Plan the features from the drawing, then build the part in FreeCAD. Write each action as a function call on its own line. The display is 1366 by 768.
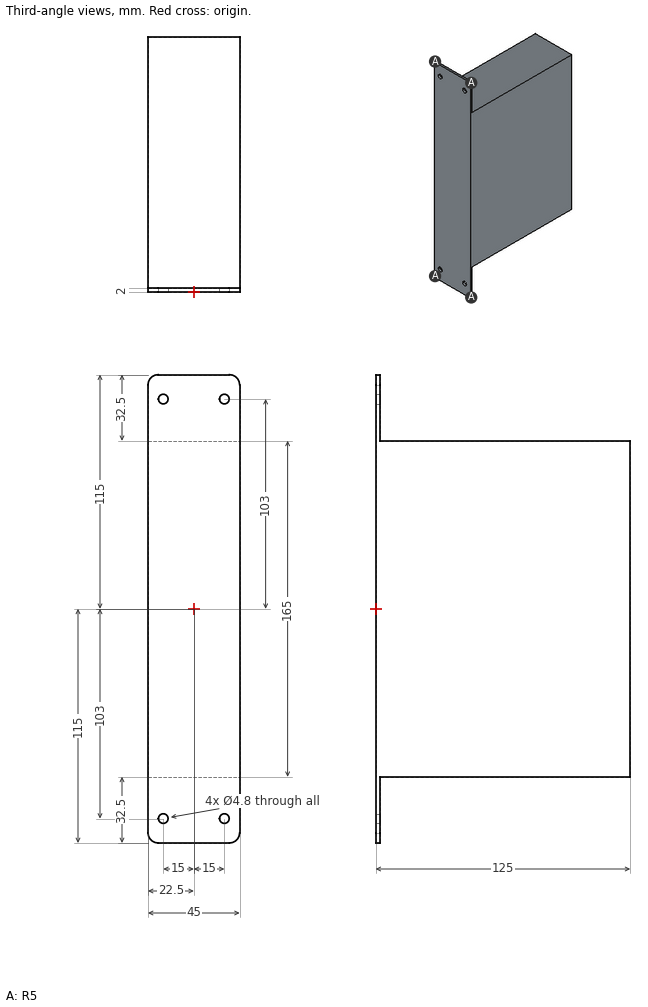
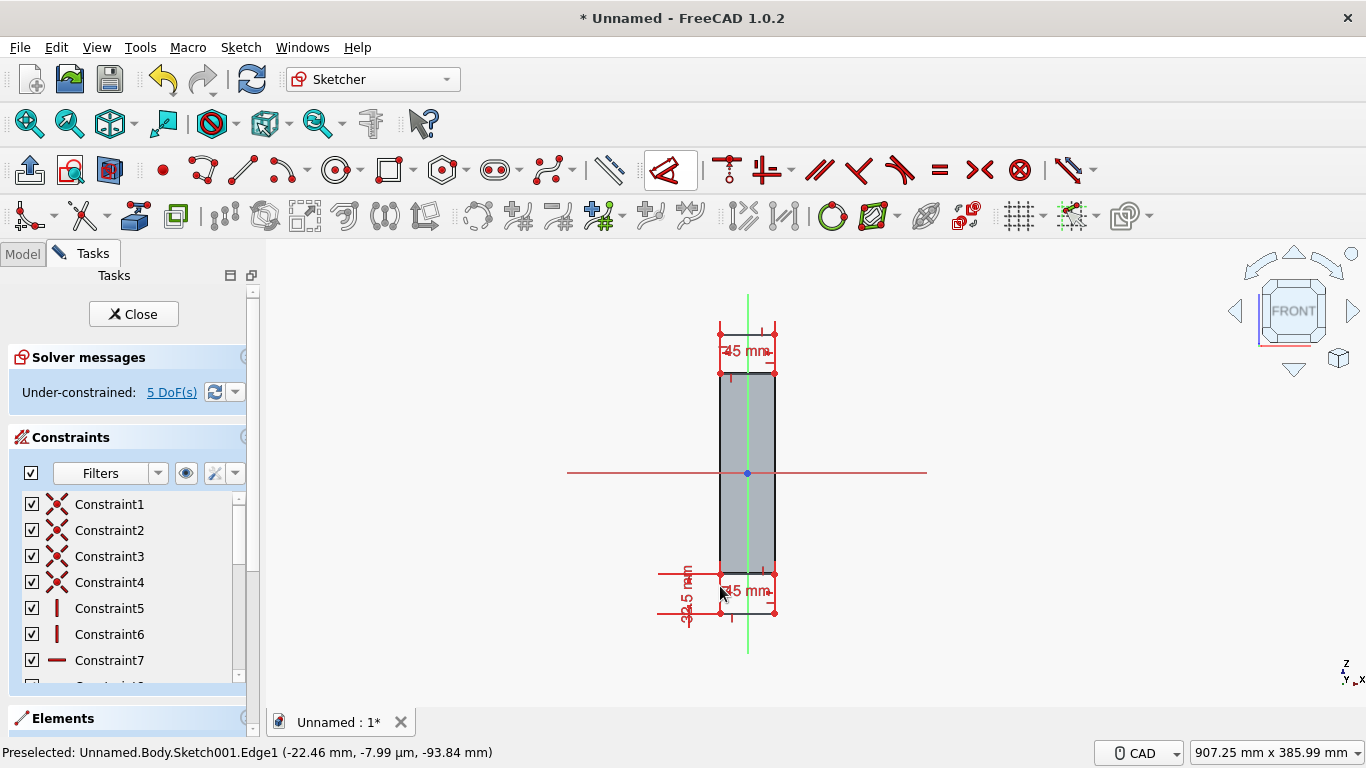
click(720, 362)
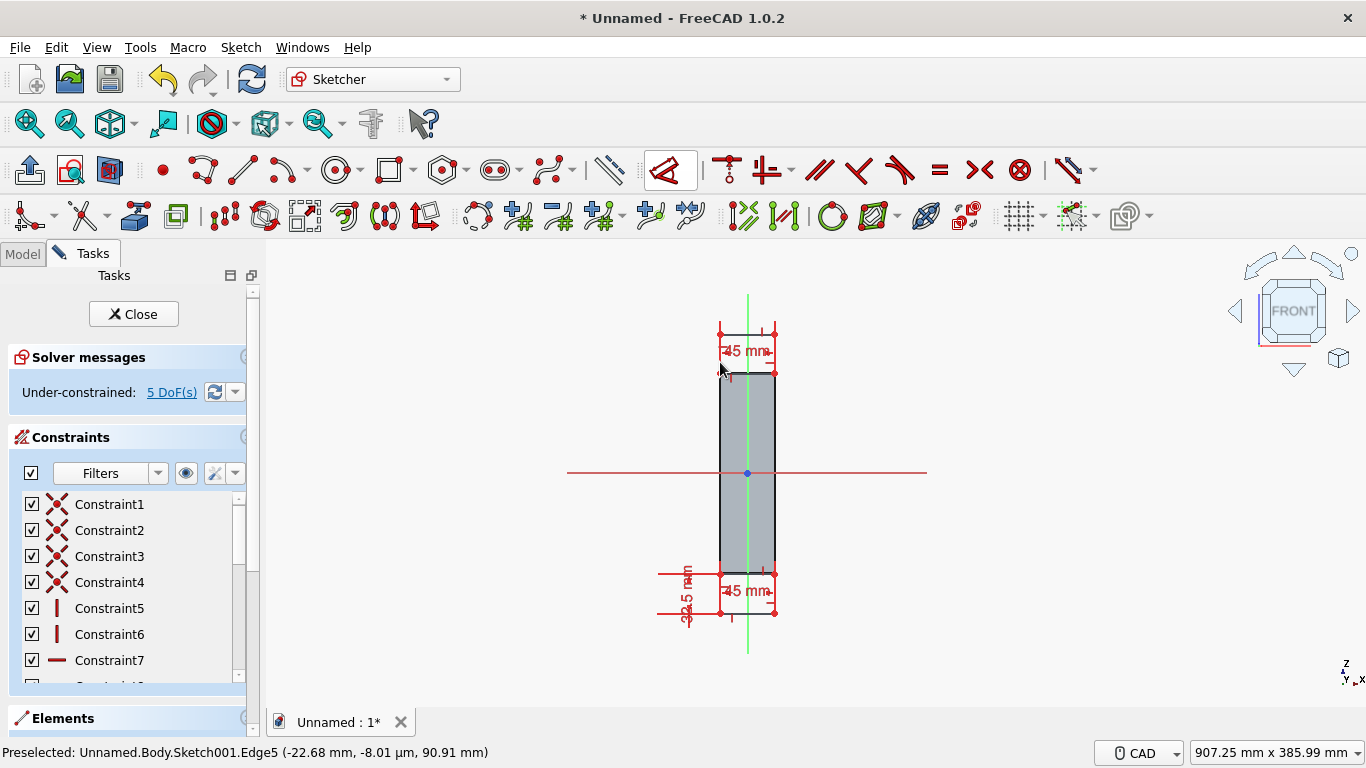
click(692, 170)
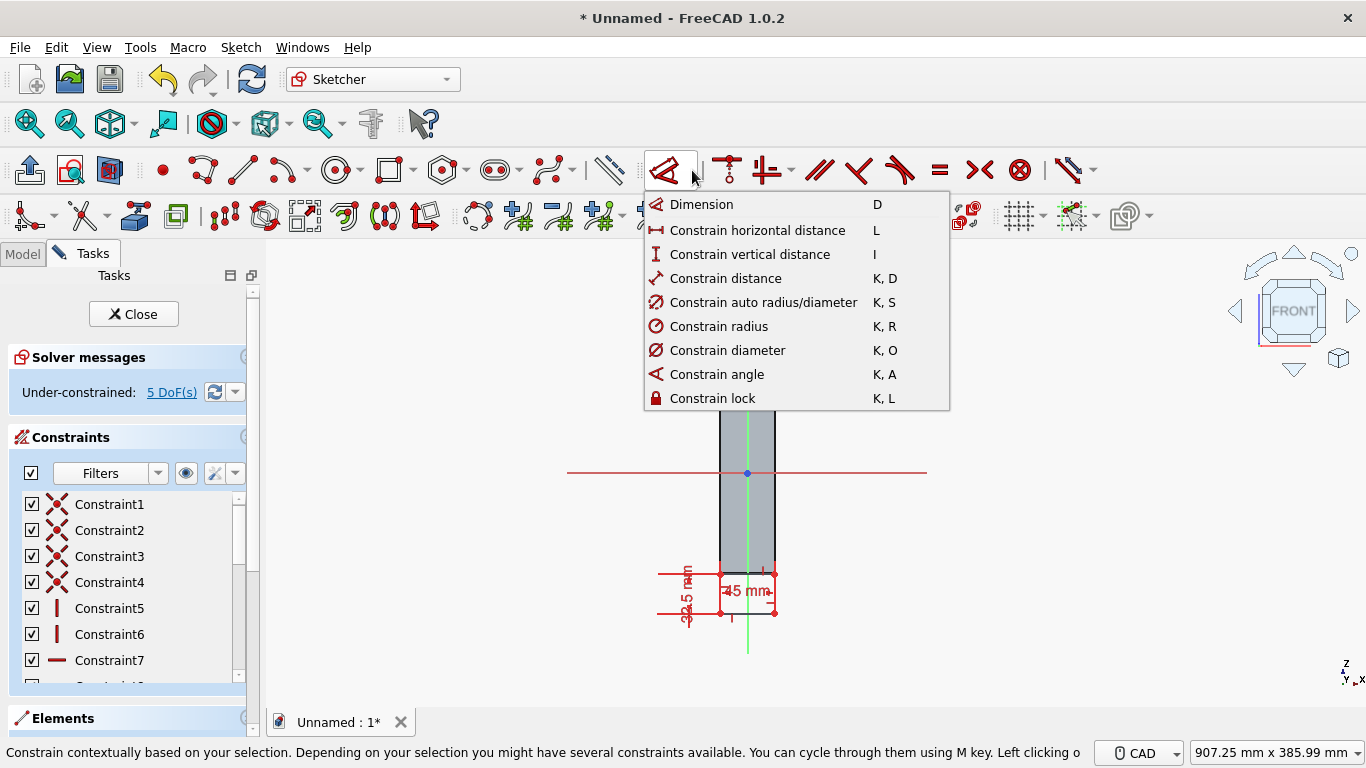
click(797, 254)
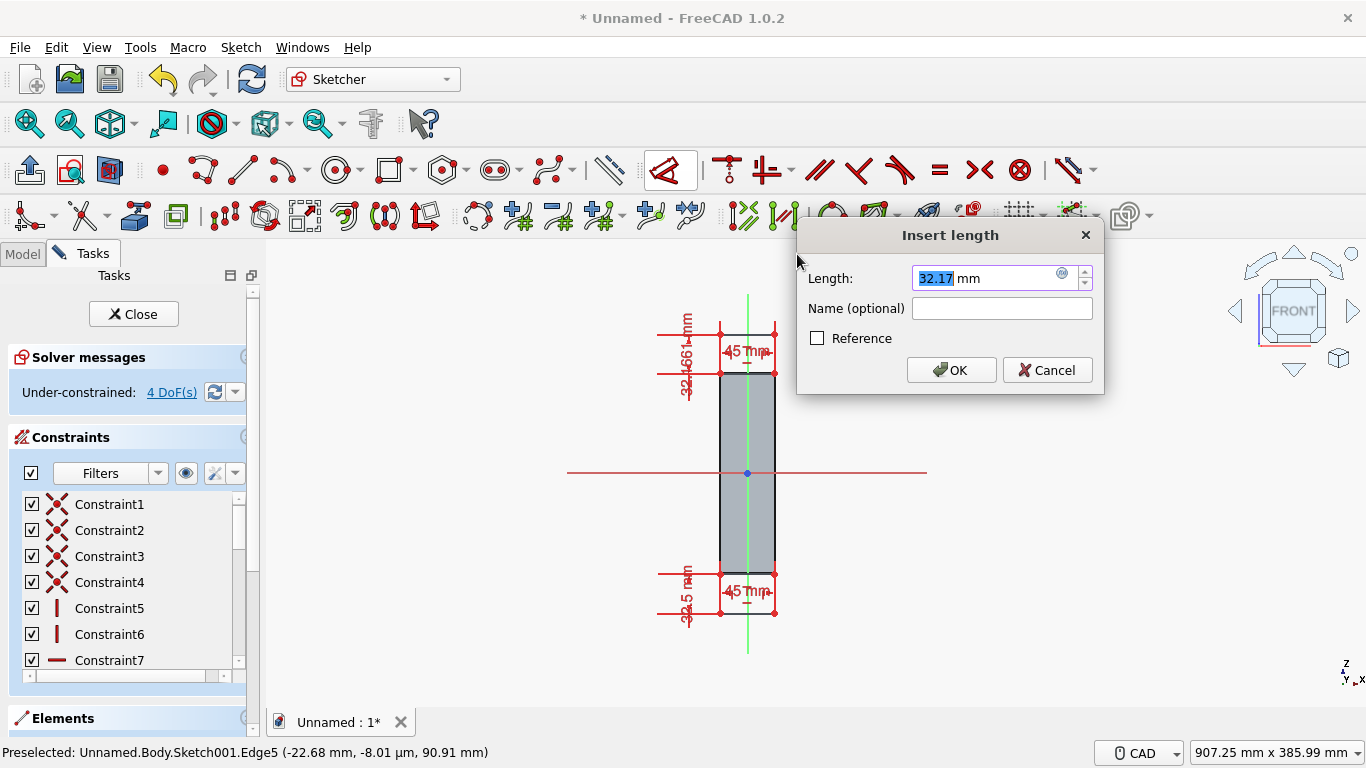
text(32.5)
key(Return)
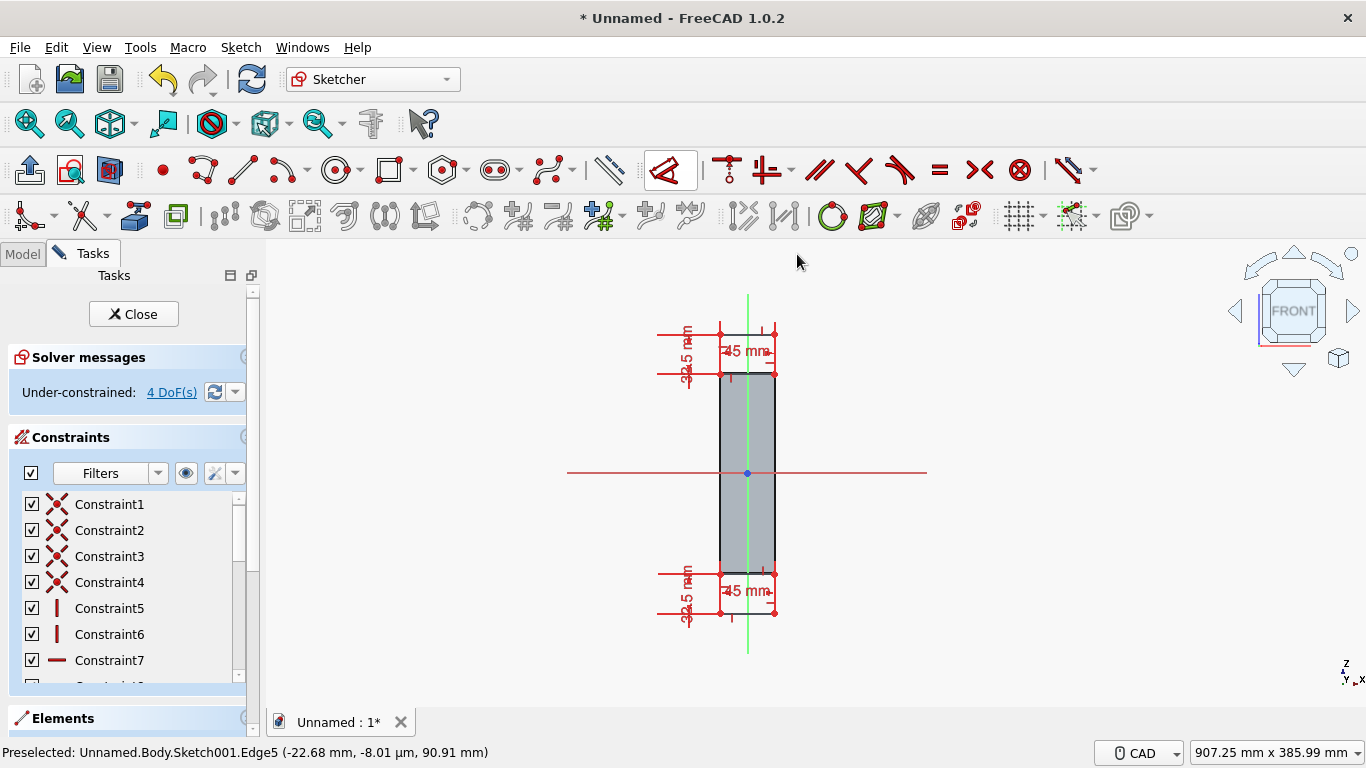
click(720, 614)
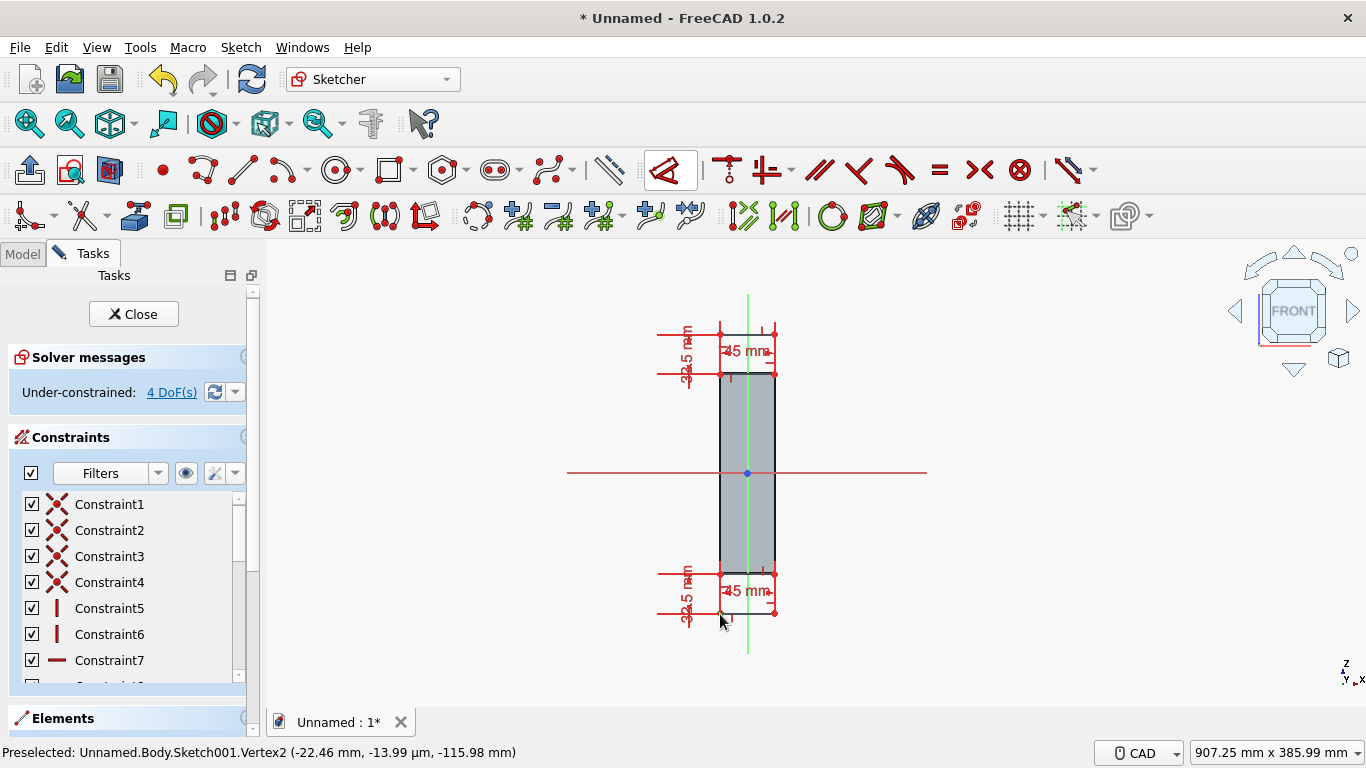
key(i)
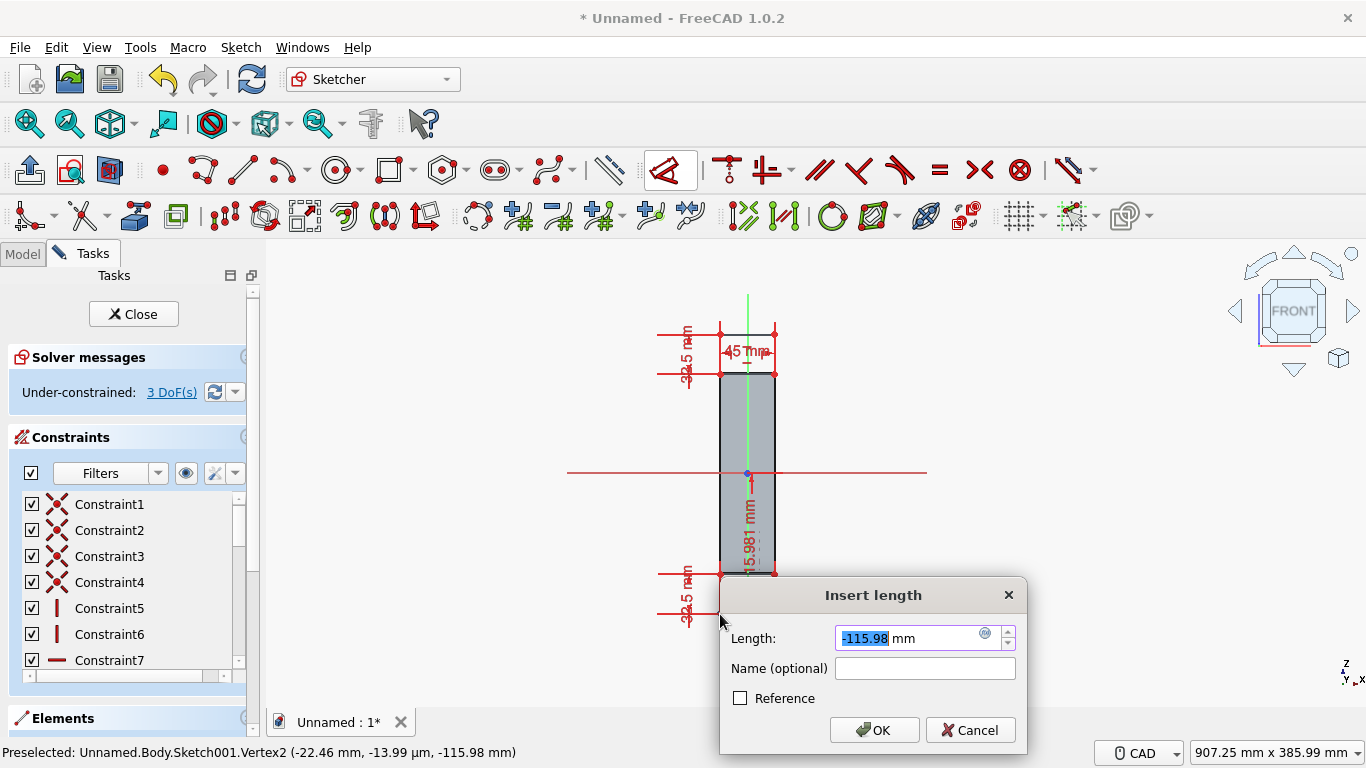
text(-115)
key(Return)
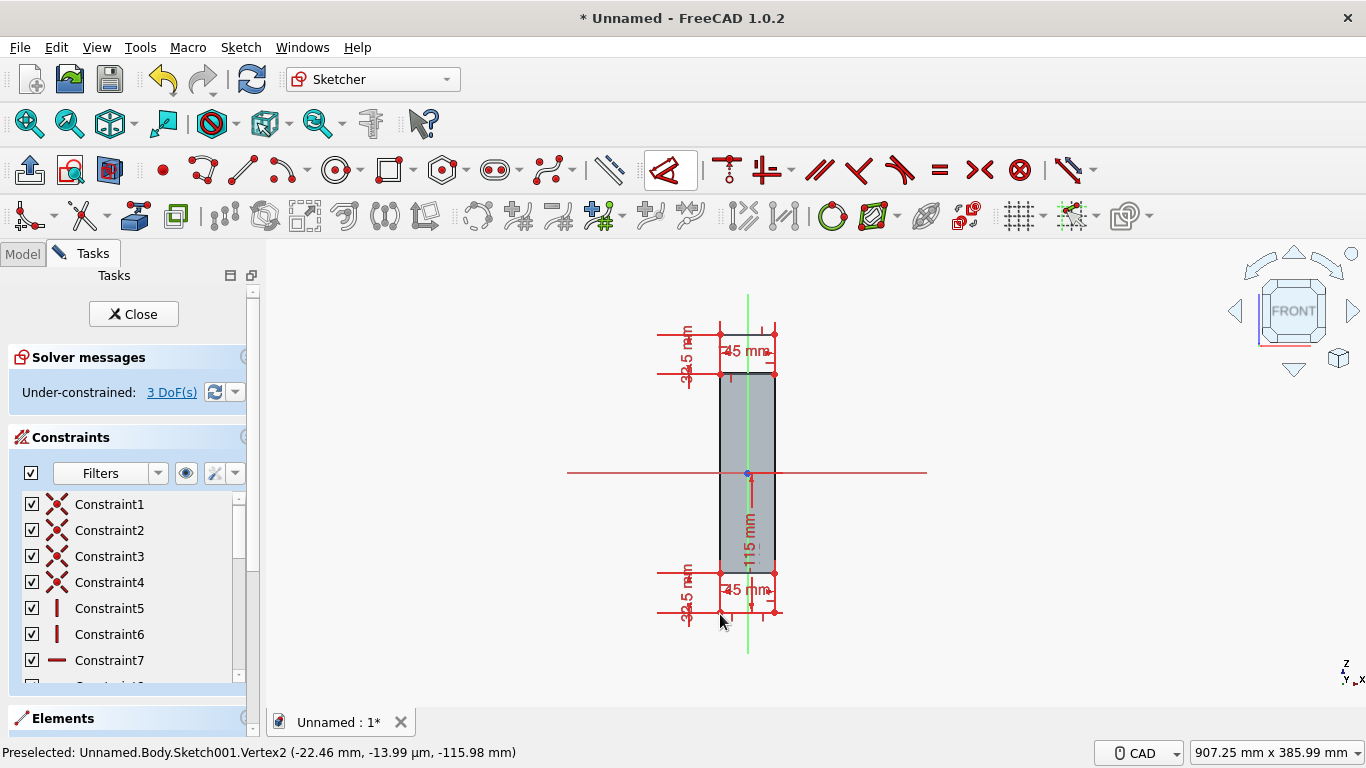
click(720, 335)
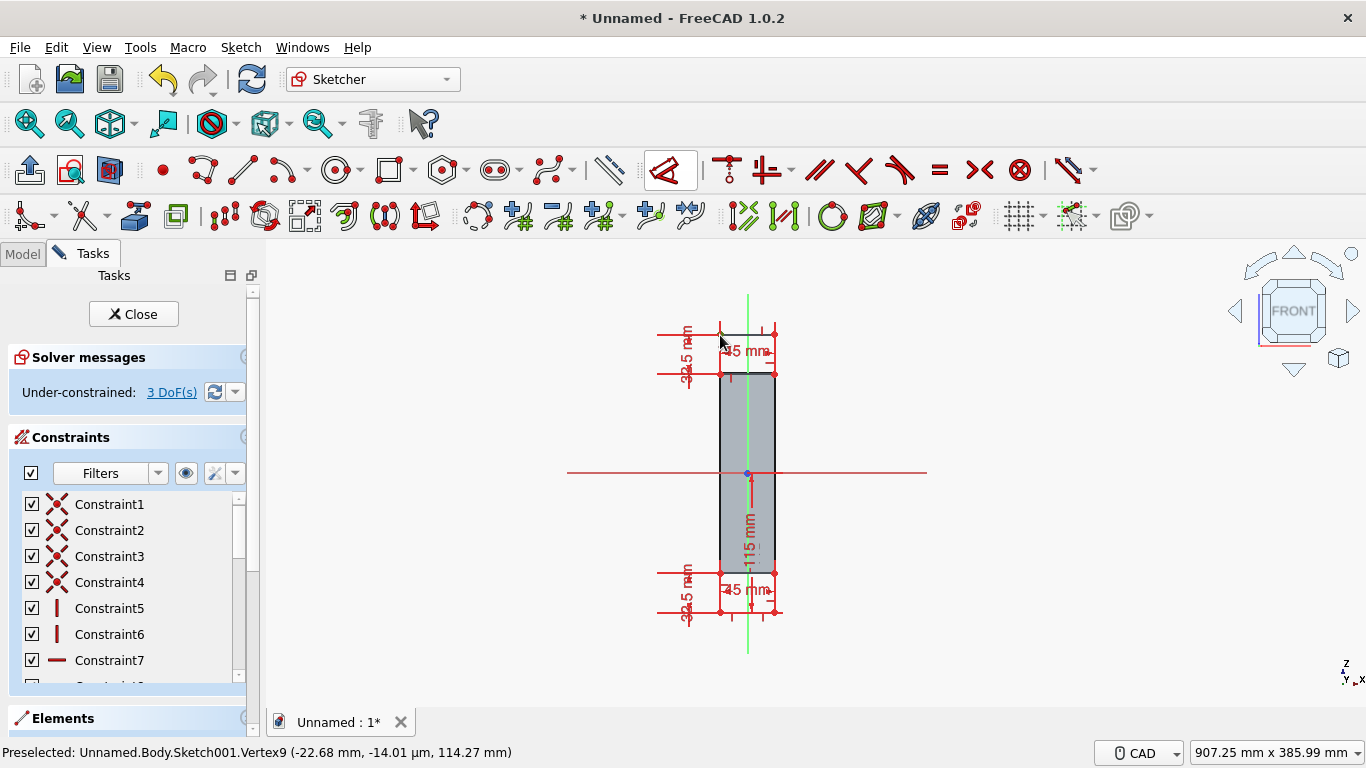
key(i)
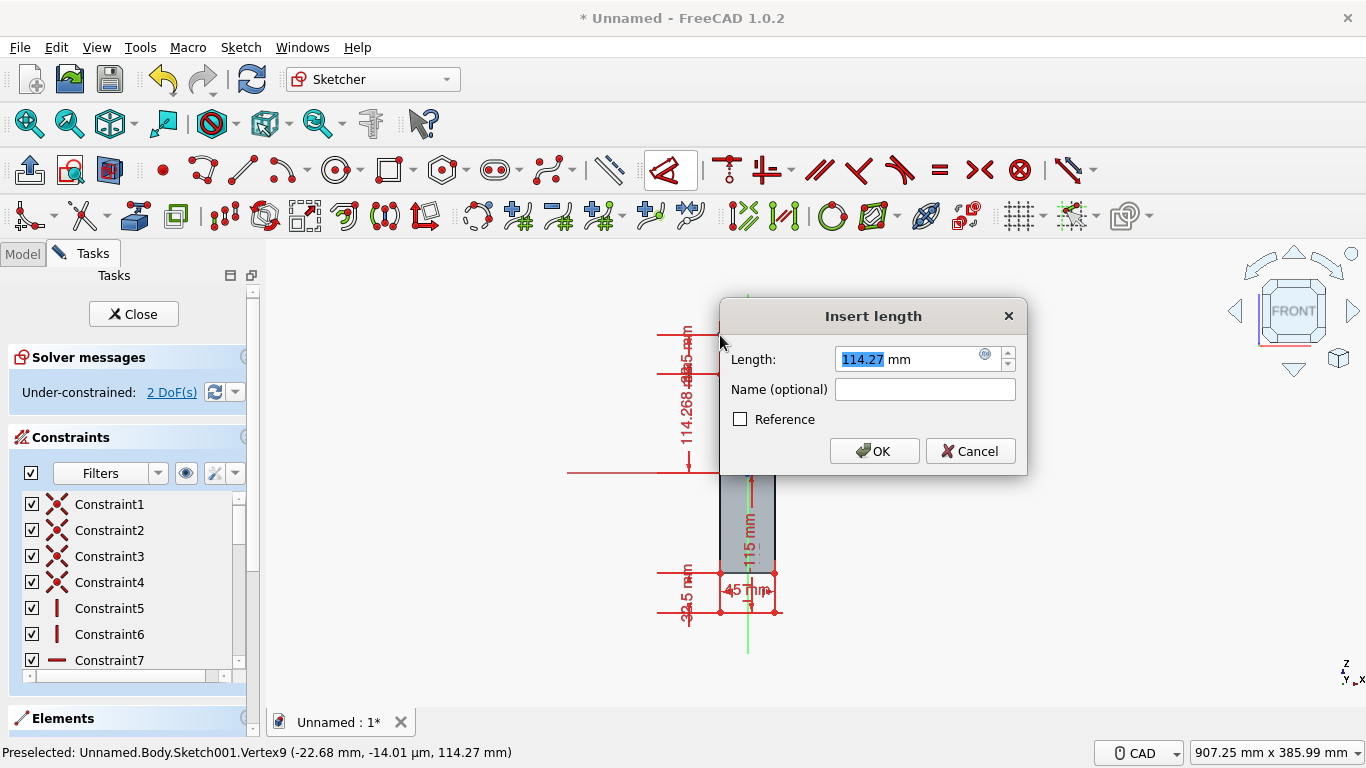
text(115)
key(Return)